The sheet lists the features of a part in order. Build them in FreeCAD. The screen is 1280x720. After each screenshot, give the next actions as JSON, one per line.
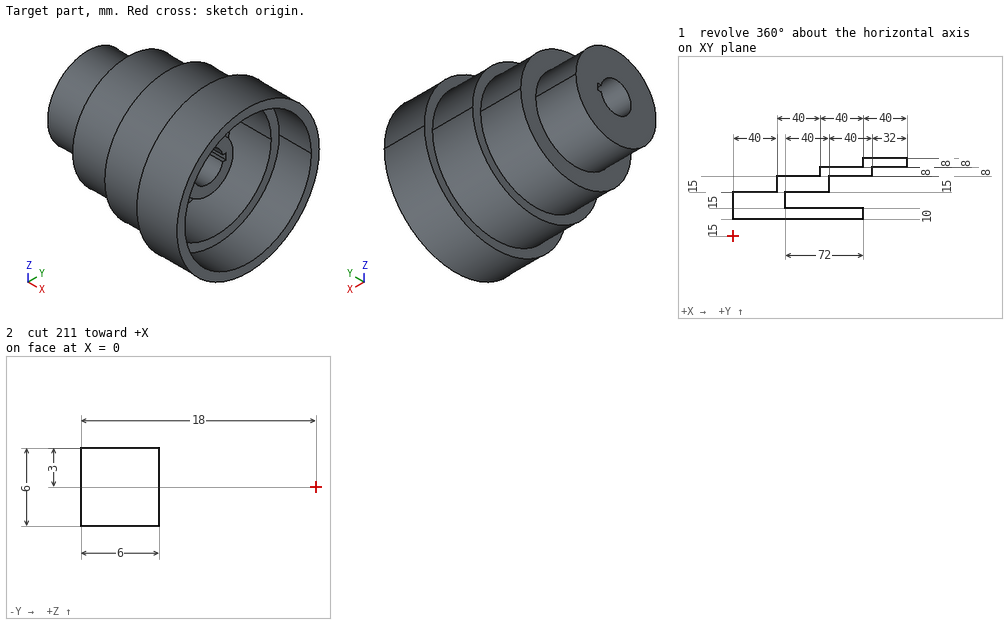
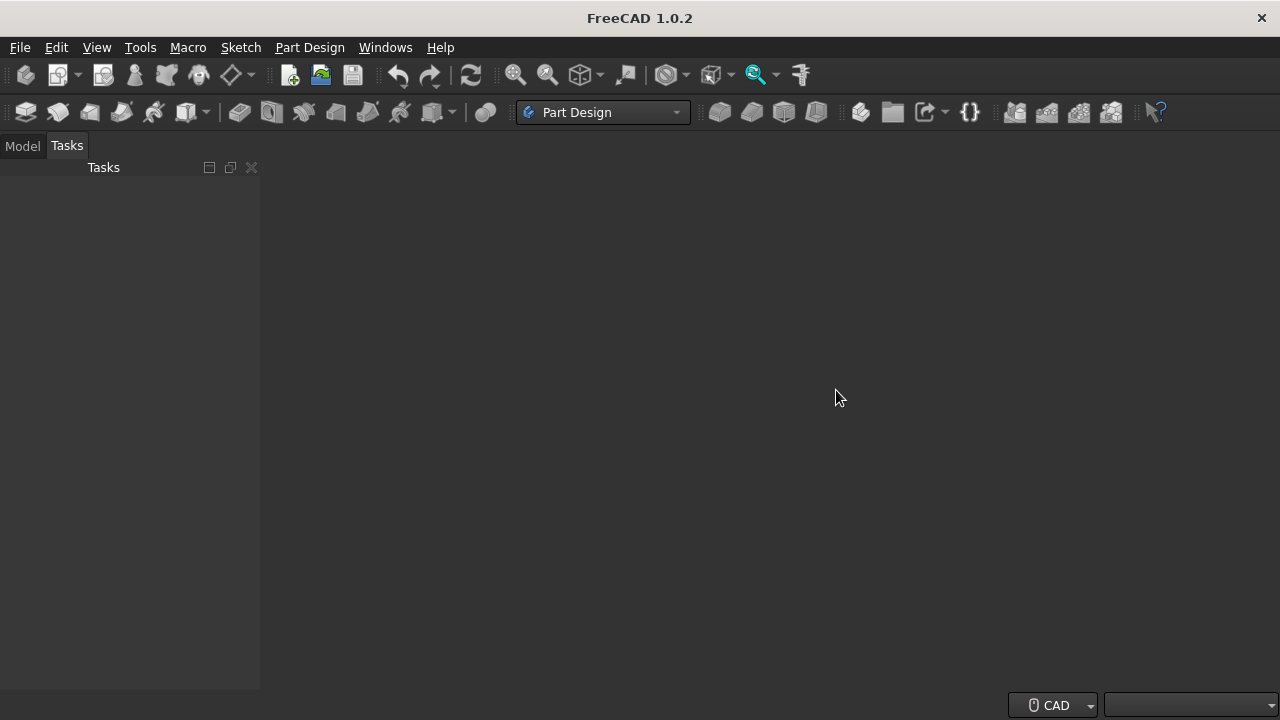
{"action": "key", "text": "ctrl+n"}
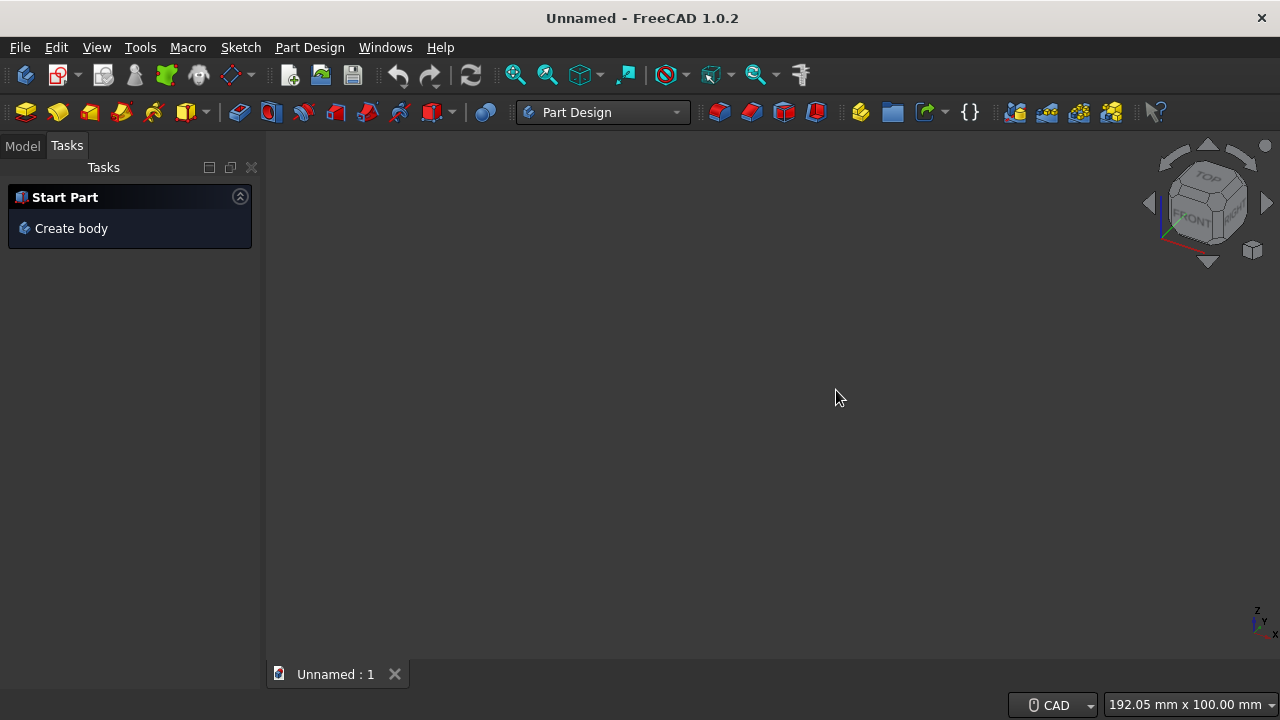
{"action": "left_click", "coordinate": [58, 76]}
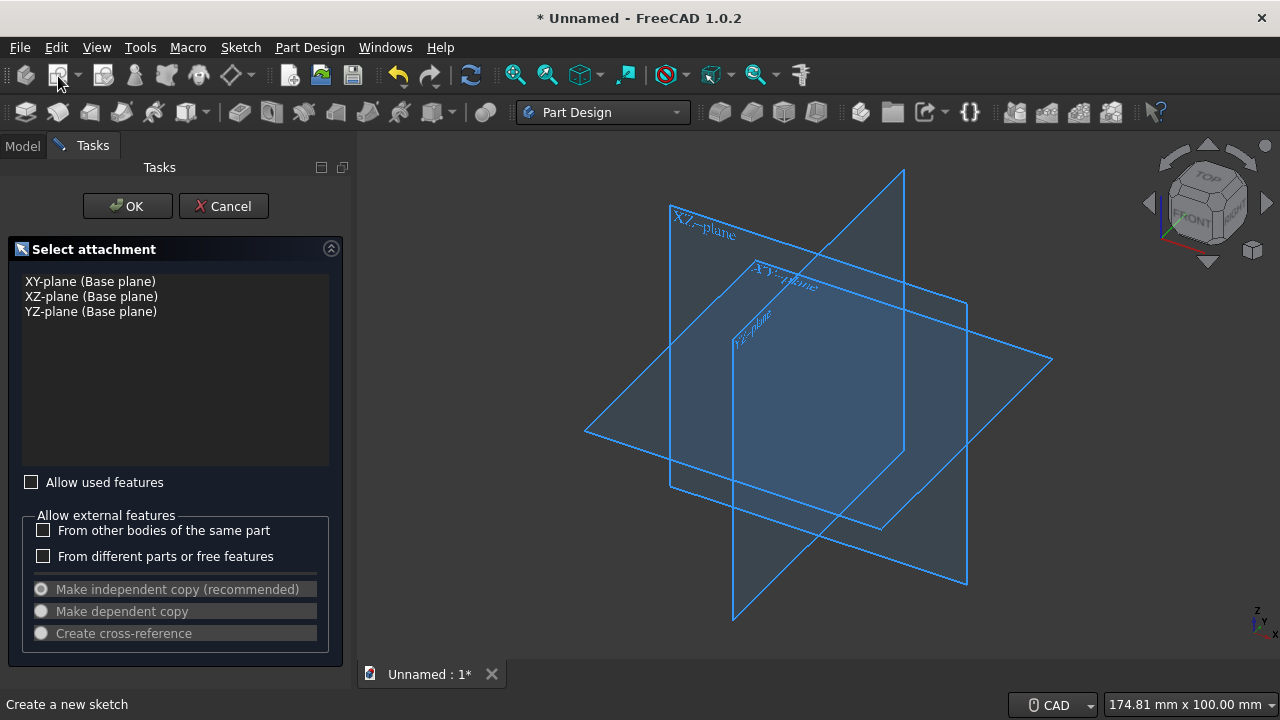
{"action": "left_click", "coordinate": [82, 282]}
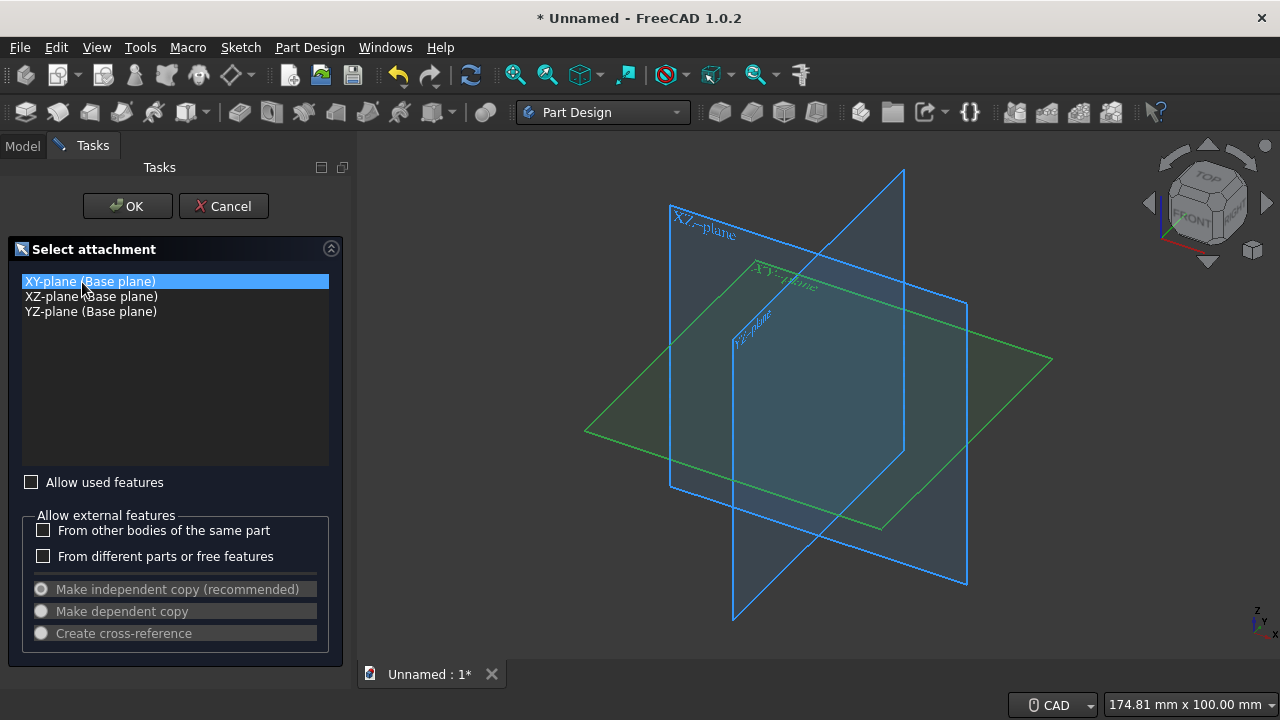
{"action": "left_click", "coordinate": [128, 206]}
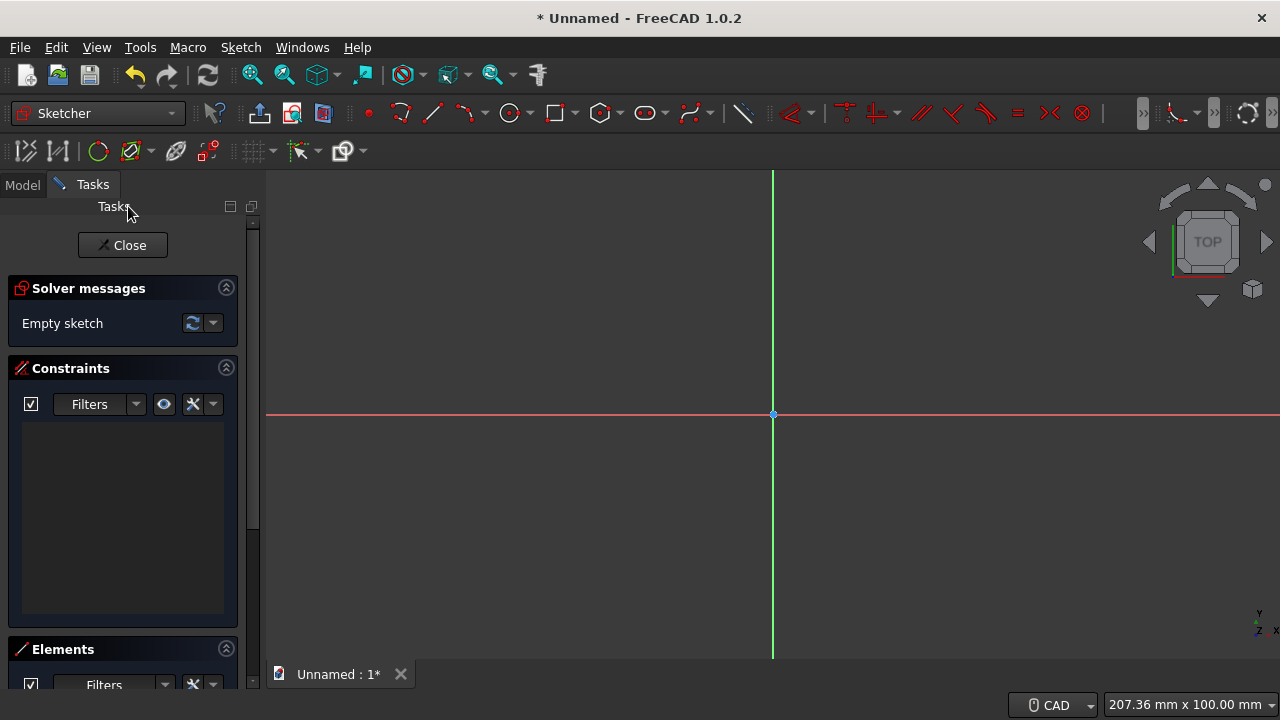
{"action": "scroll", "coordinate": [294, 626], "scroll_direction": "down", "scroll_amount": 3}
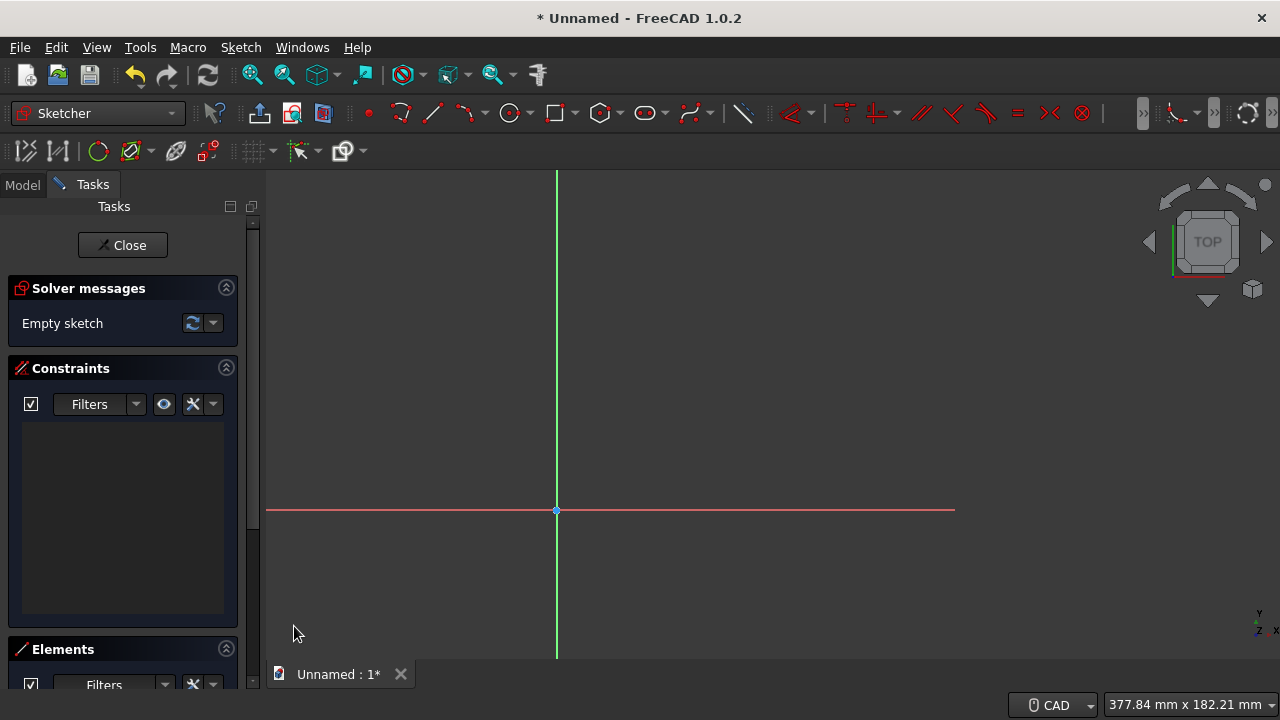
{"action": "key", "text": "g m"}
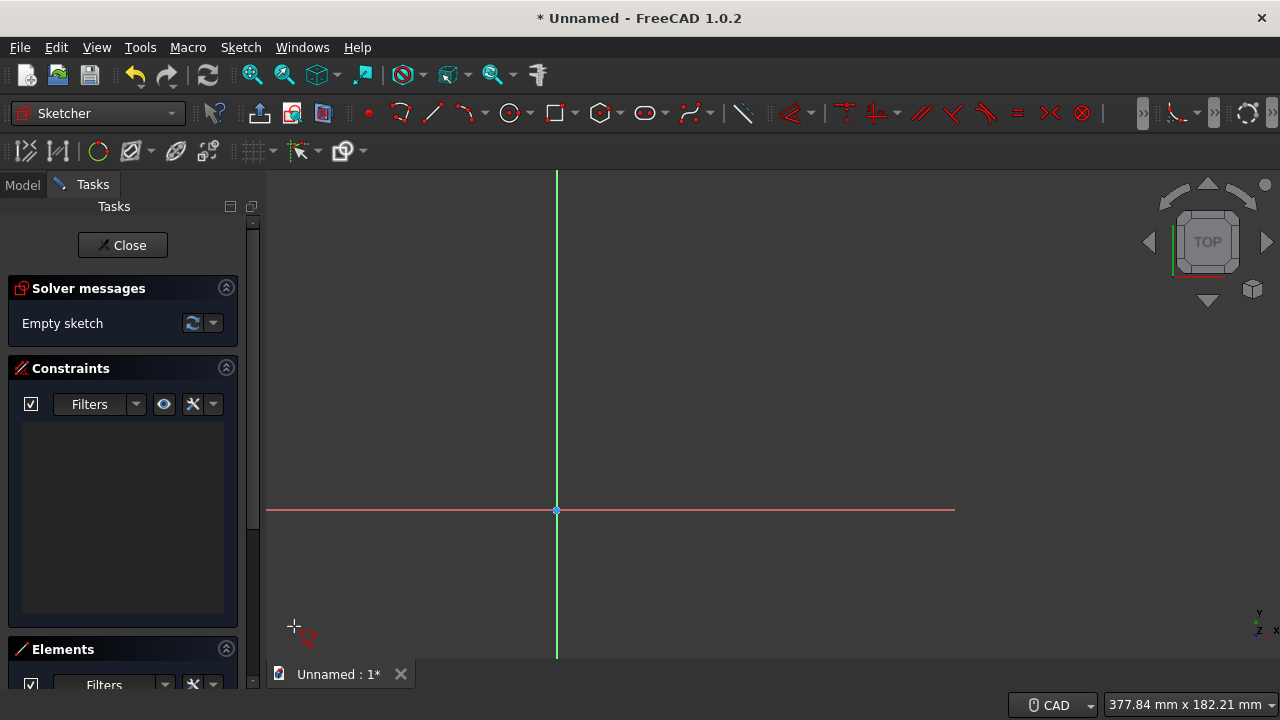
{"action": "left_click", "coordinate": [557, 470]}
{"action": "left_click", "coordinate": [879, 470]}
{"action": "left_click", "coordinate": [879, 443]}
{"action": "left_click", "coordinate": [686, 443]}
{"action": "left_click", "coordinate": [686, 403]}
{"action": "left_click", "coordinate": [793, 403]}
{"action": "left_click", "coordinate": [793, 363]}
{"action": "left_click", "coordinate": [900, 363]}
{"action": "left_click", "coordinate": [900, 341]}
{"action": "left_click", "coordinate": [986, 341]}
{"action": "left_click", "coordinate": [986, 320]}
{"action": "left_click", "coordinate": [879, 320]}
{"action": "left_click", "coordinate": [879, 341]}
{"action": "left_click", "coordinate": [772, 341]}
{"action": "left_click", "coordinate": [772, 363]}
{"action": "left_click", "coordinate": [664, 363]}
{"action": "left_click", "coordinate": [664, 403]}
{"action": "left_click", "coordinate": [566, 403]}
{"action": "left_click", "coordinate": [557, 471]}
{"action": "key", "text": "Escape"}
{"action": "key", "text": "Escape"}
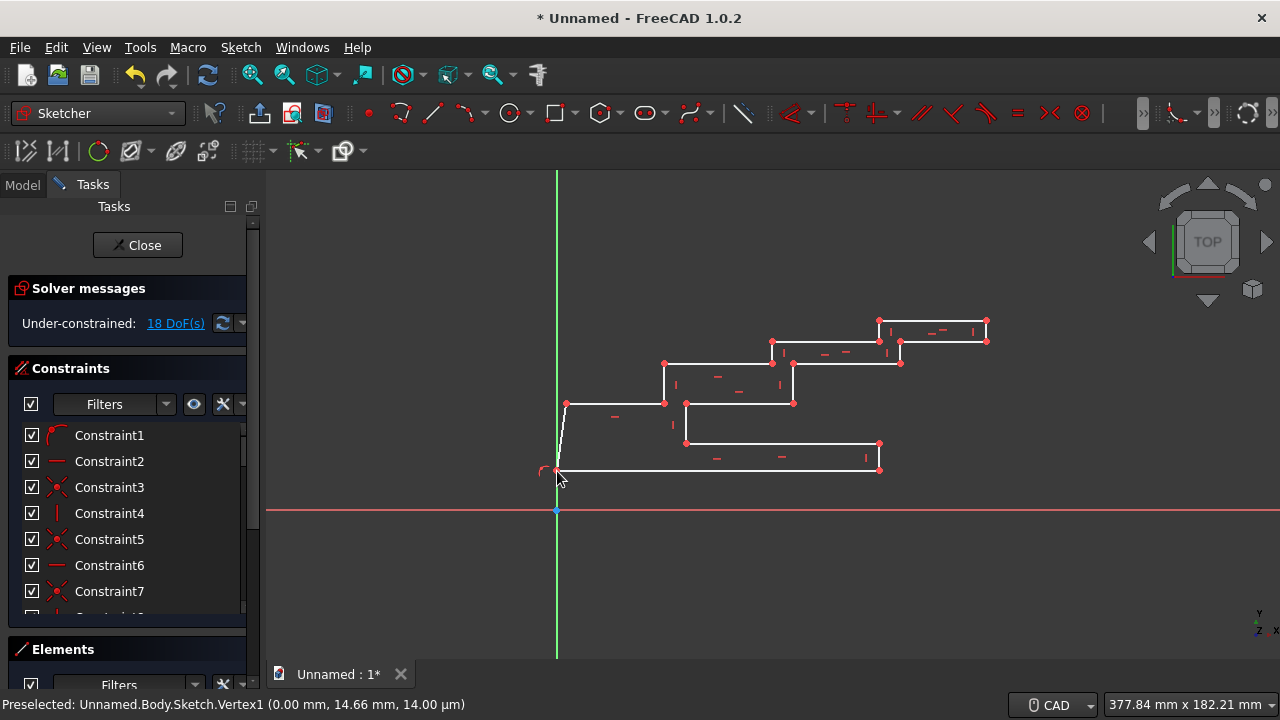
{"action": "left_click", "coordinate": [560, 451]}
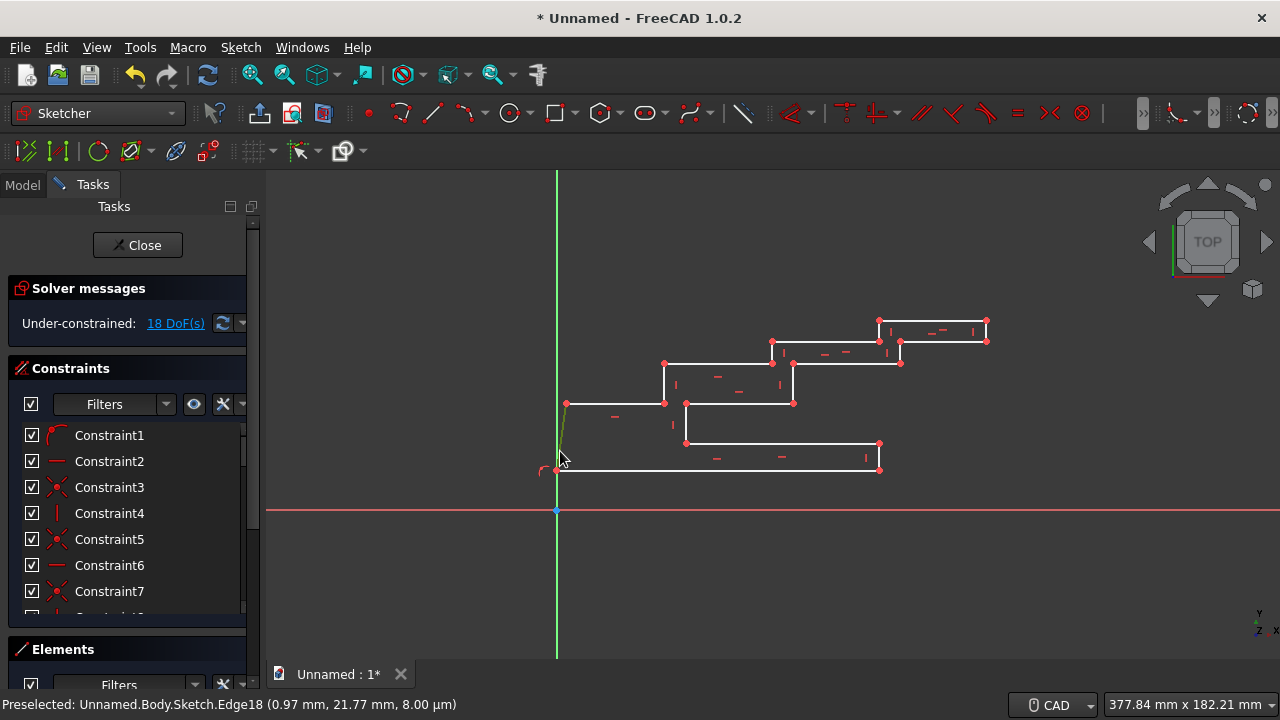
{"action": "left_click", "coordinate": [900, 114]}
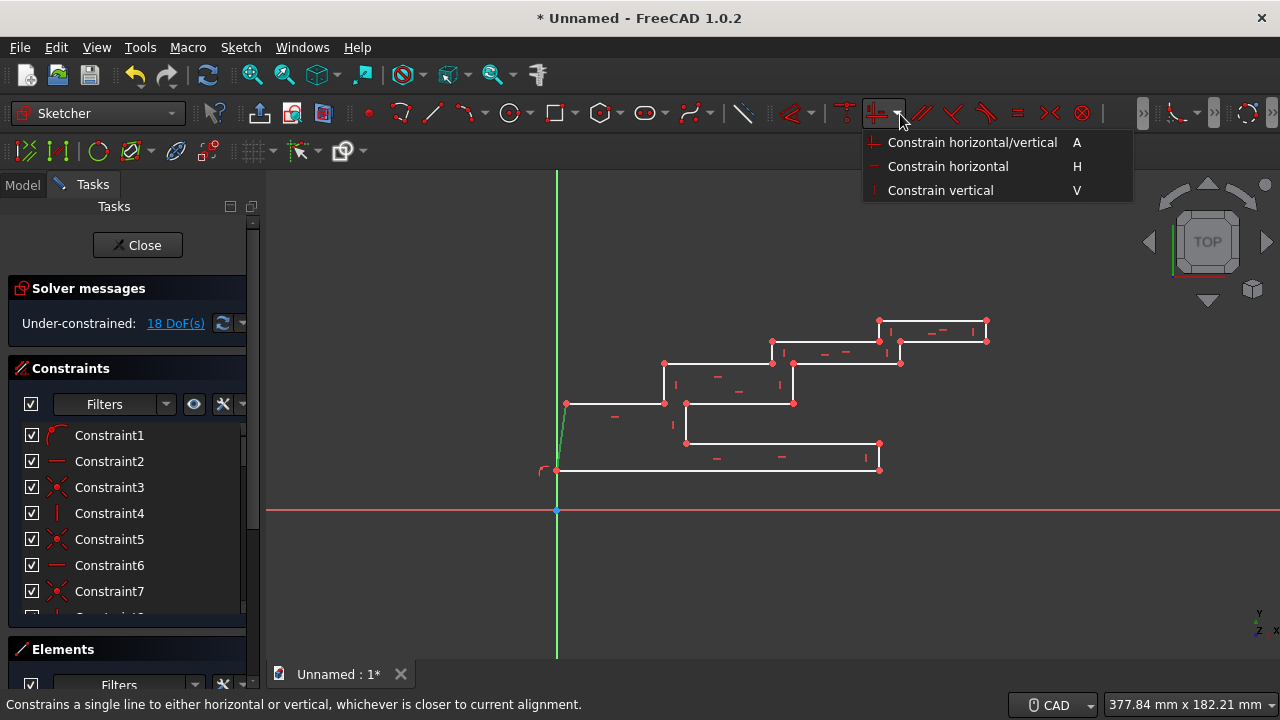
{"action": "left_click", "coordinate": [998, 190]}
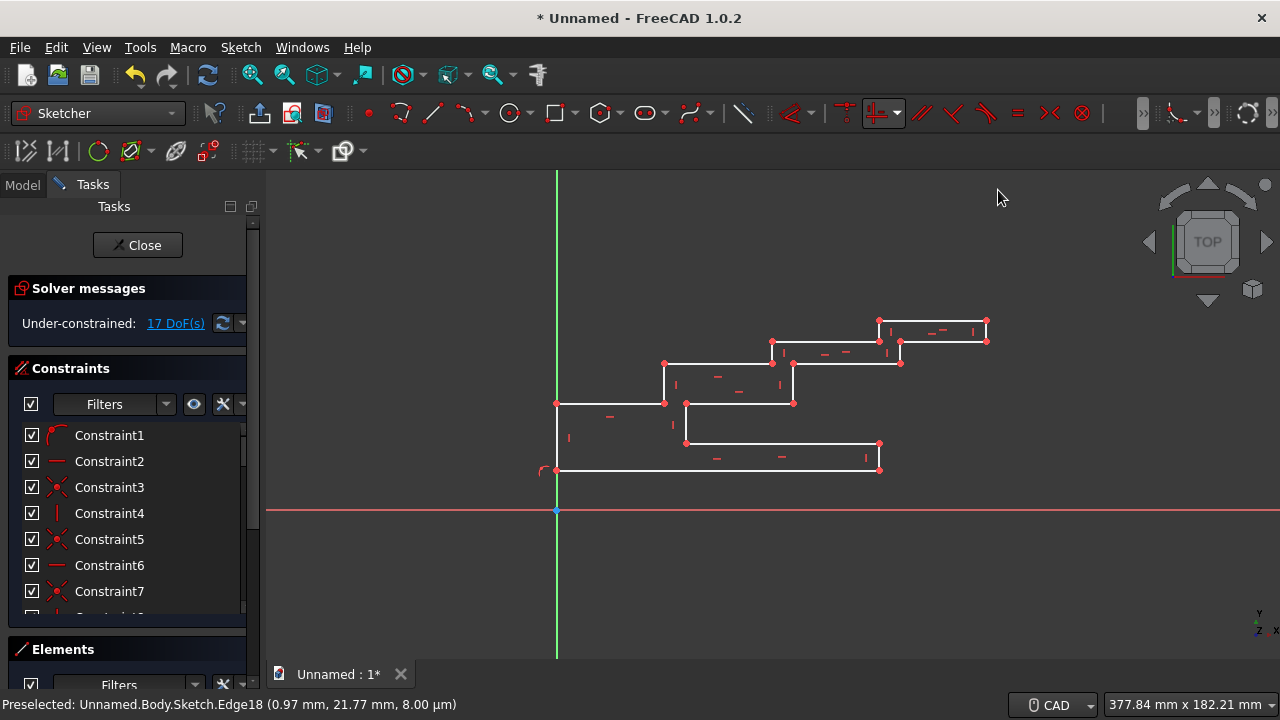
{"action": "key", "text": "d"}